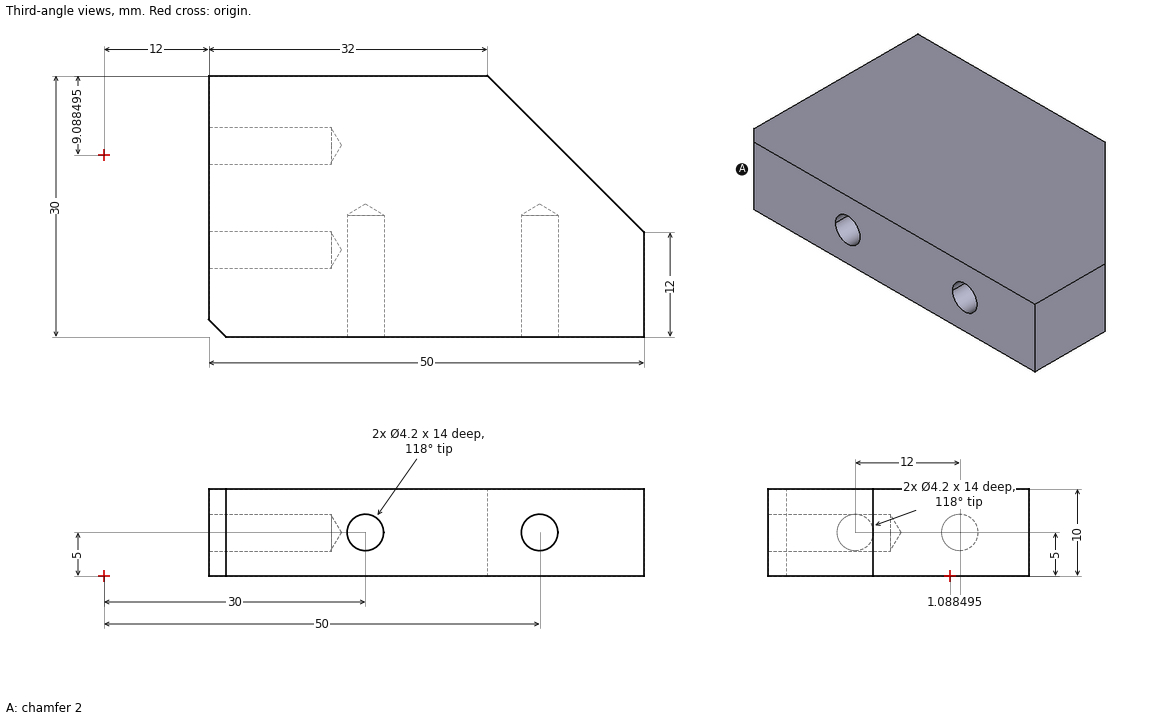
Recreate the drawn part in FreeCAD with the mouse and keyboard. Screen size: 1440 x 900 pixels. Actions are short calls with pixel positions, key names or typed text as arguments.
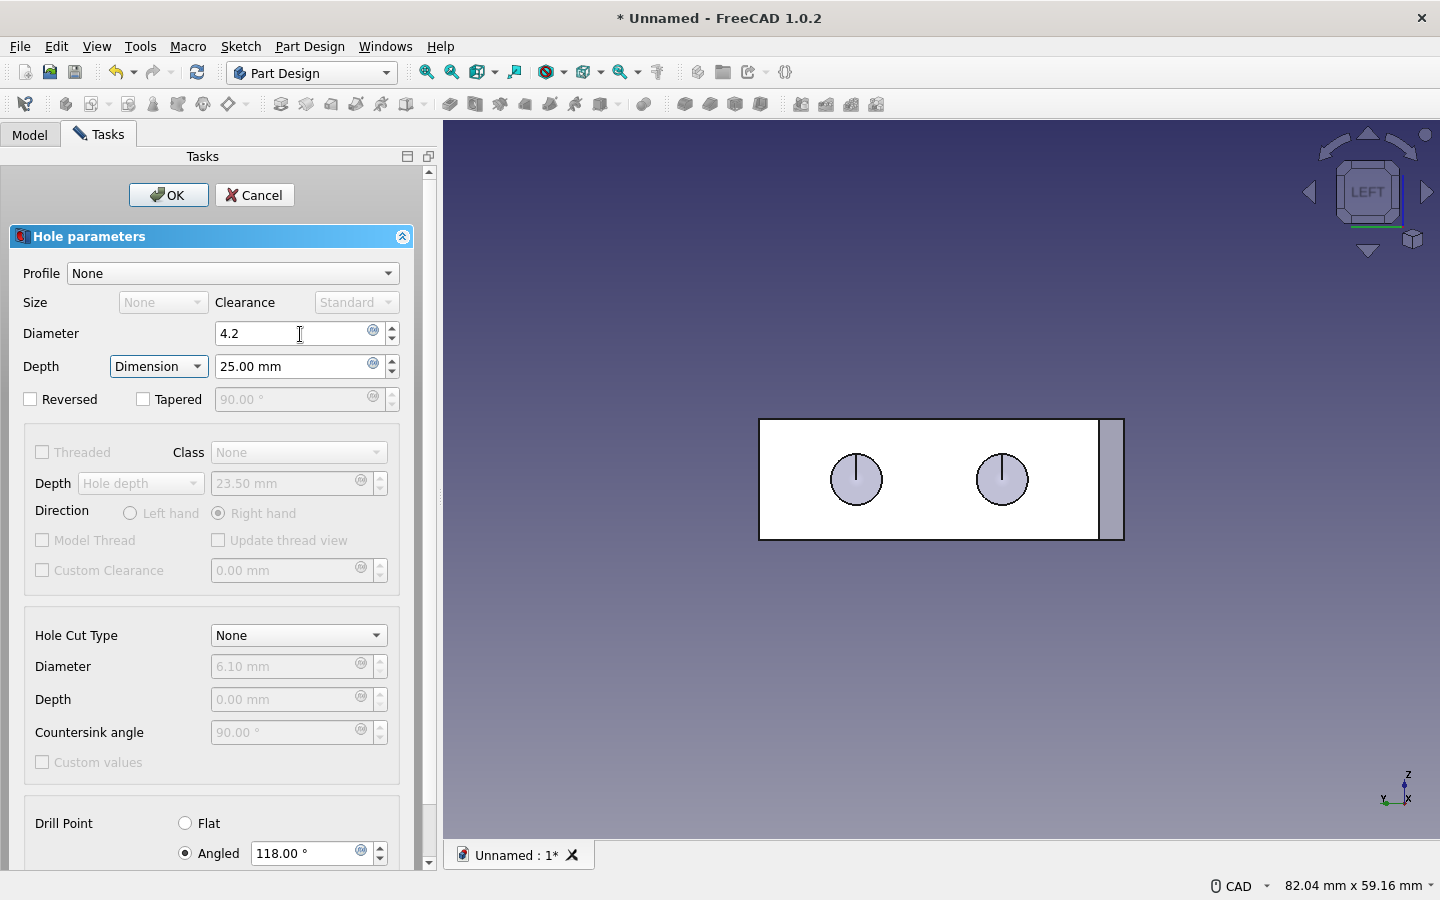
triple_click(300, 366)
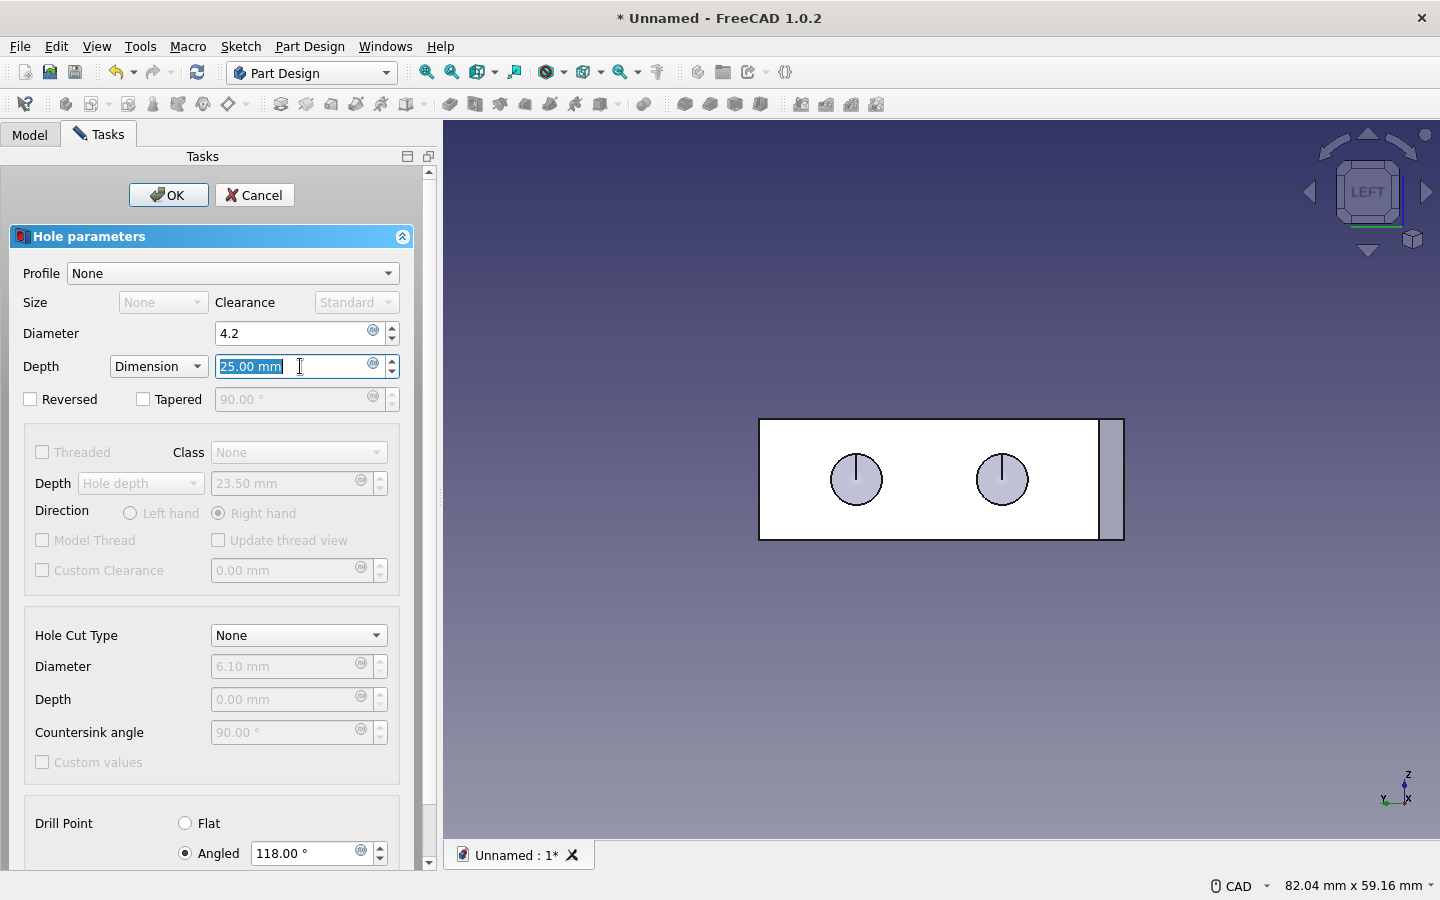
text(14)
key(Tab)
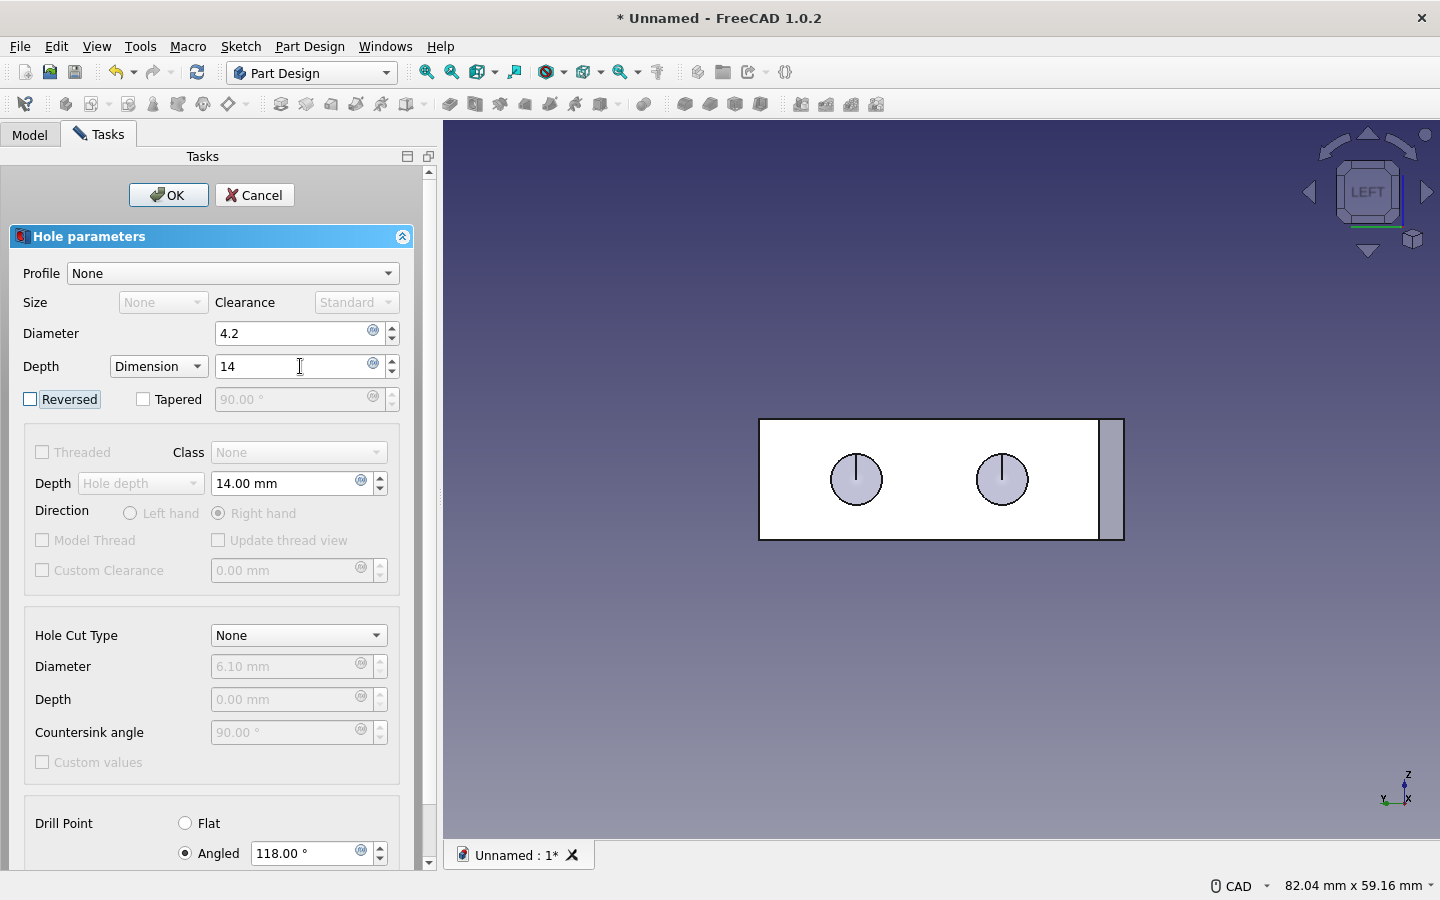
click(169, 195)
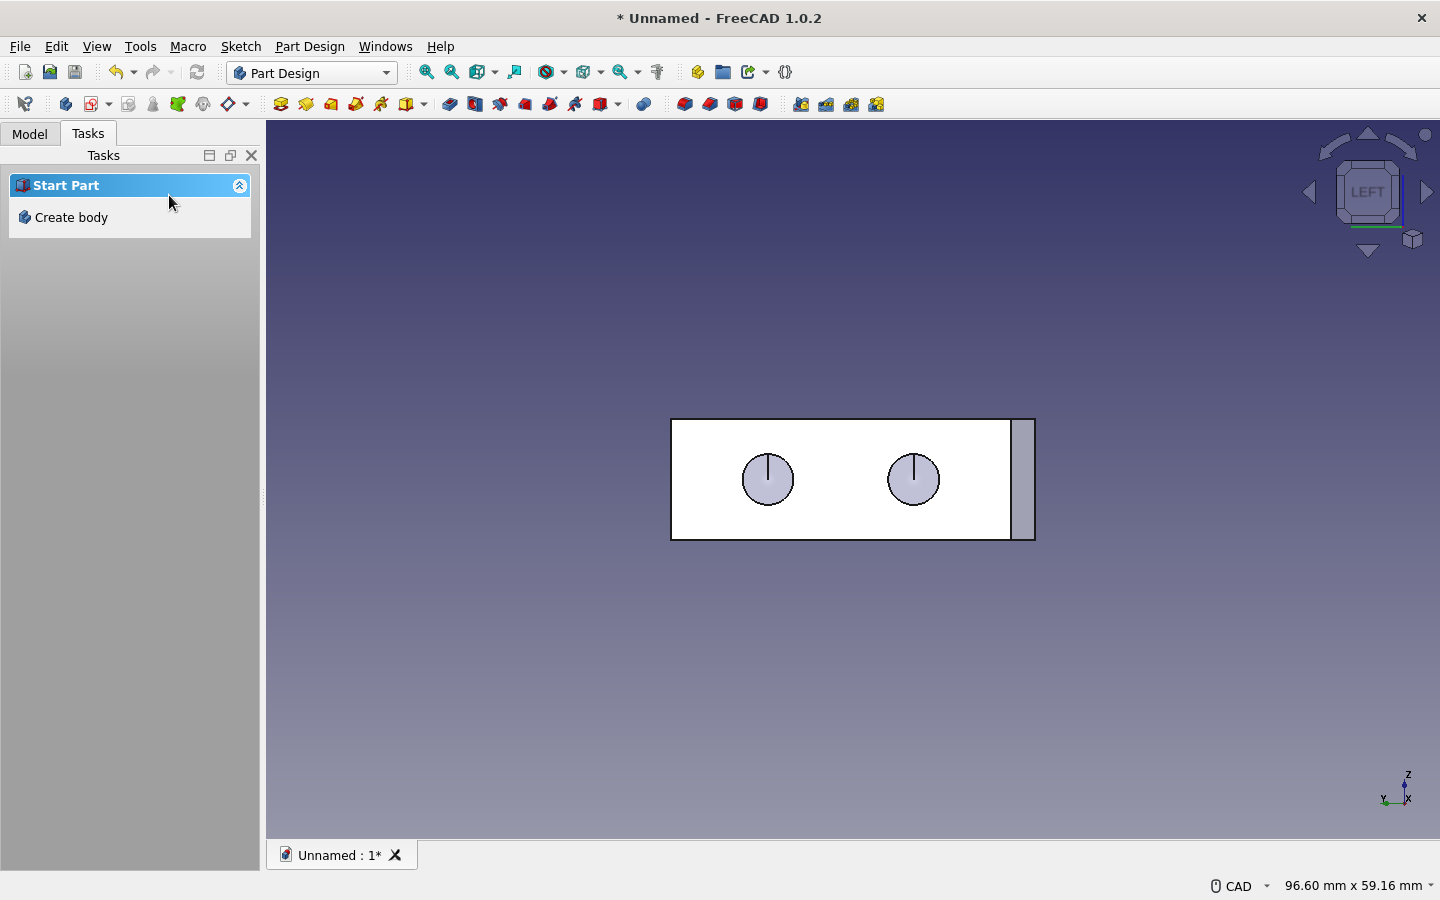
click(427, 72)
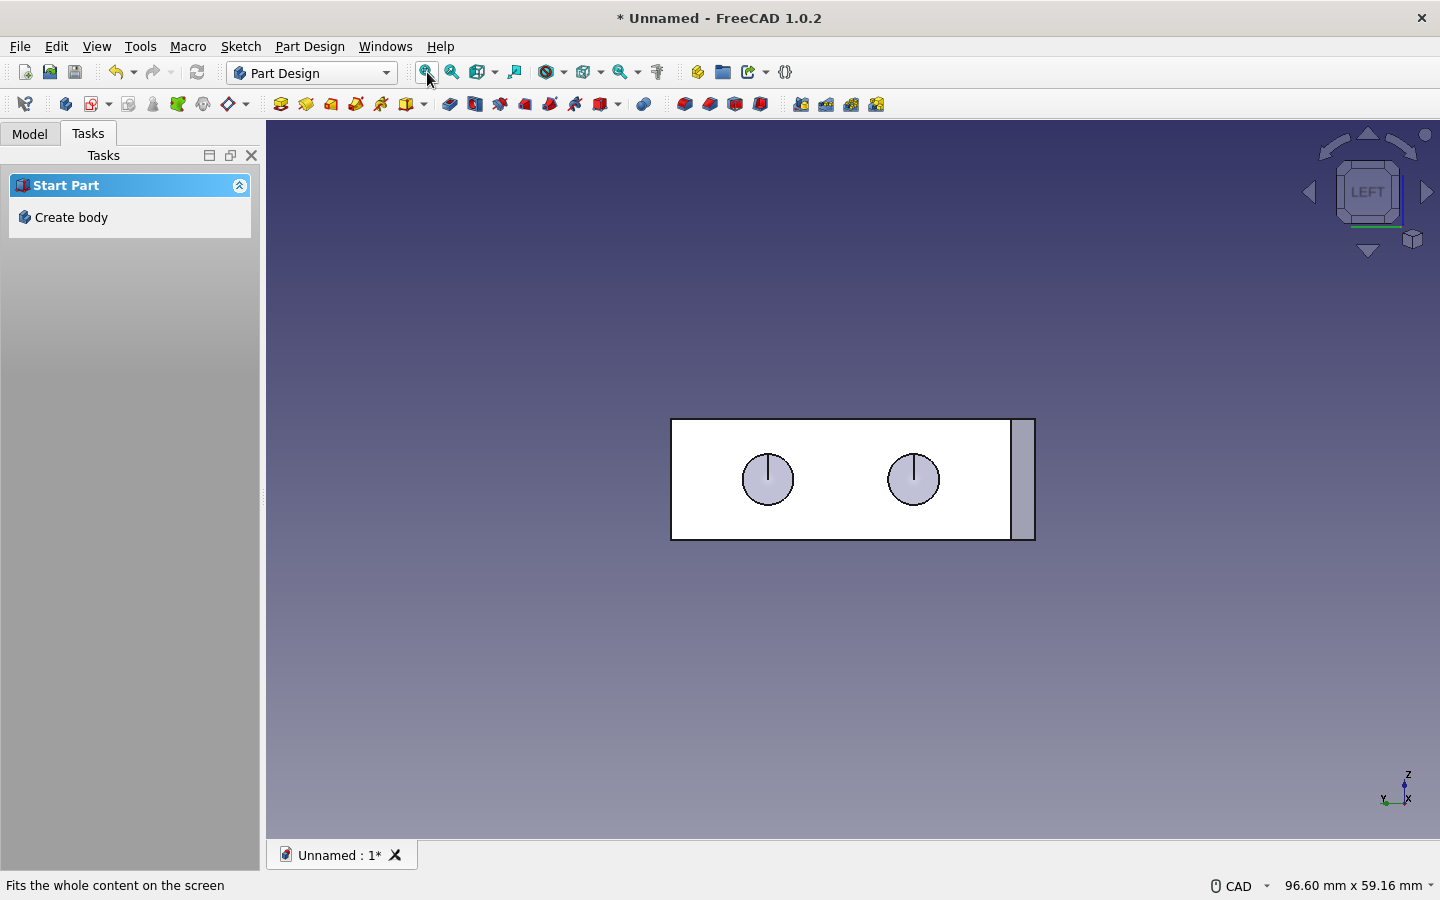
key(0)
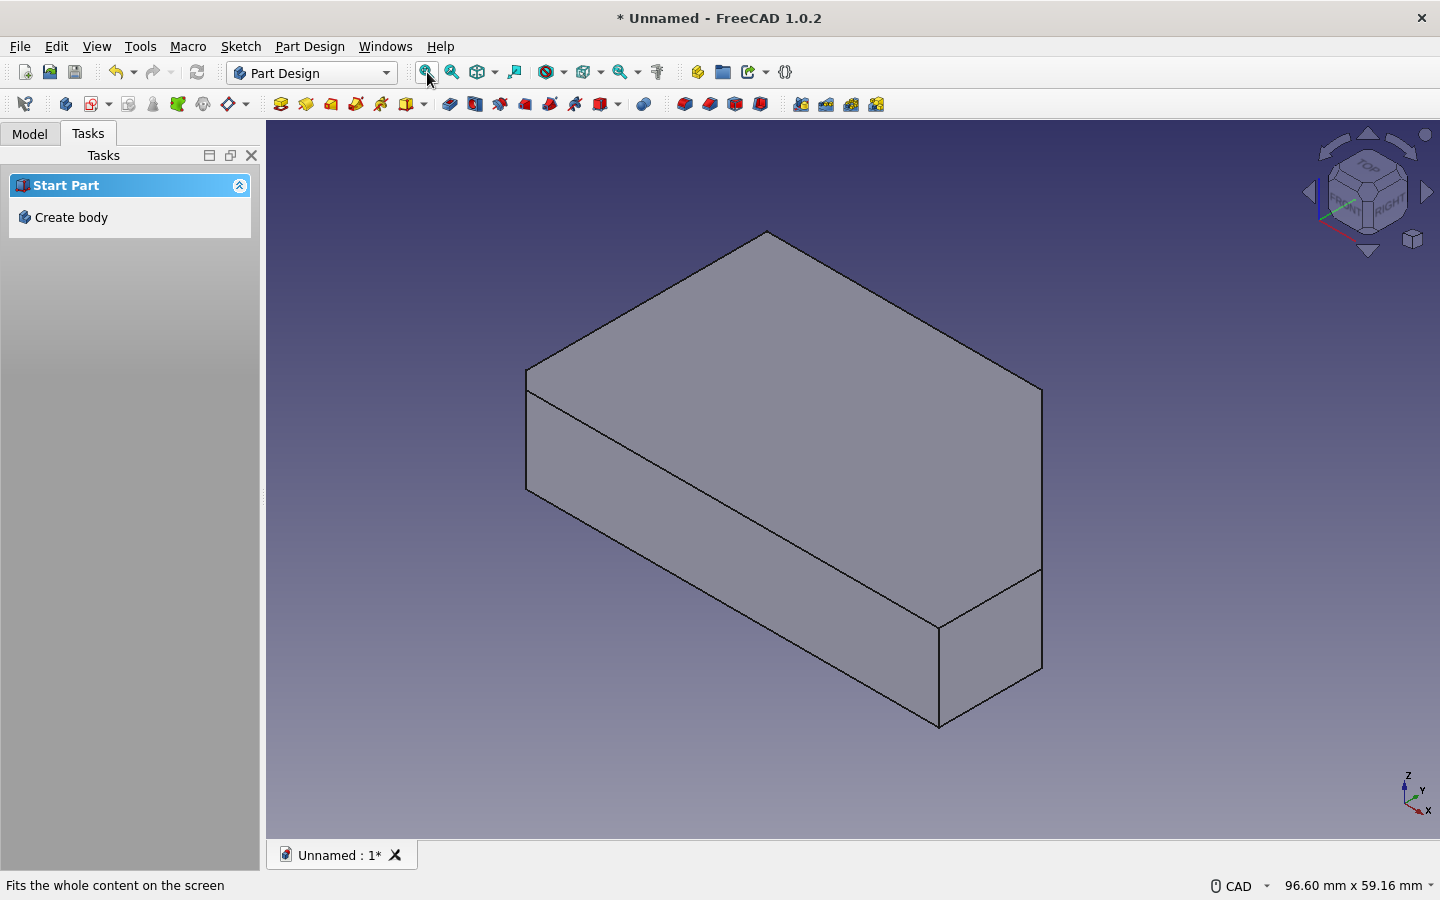
click(851, 626)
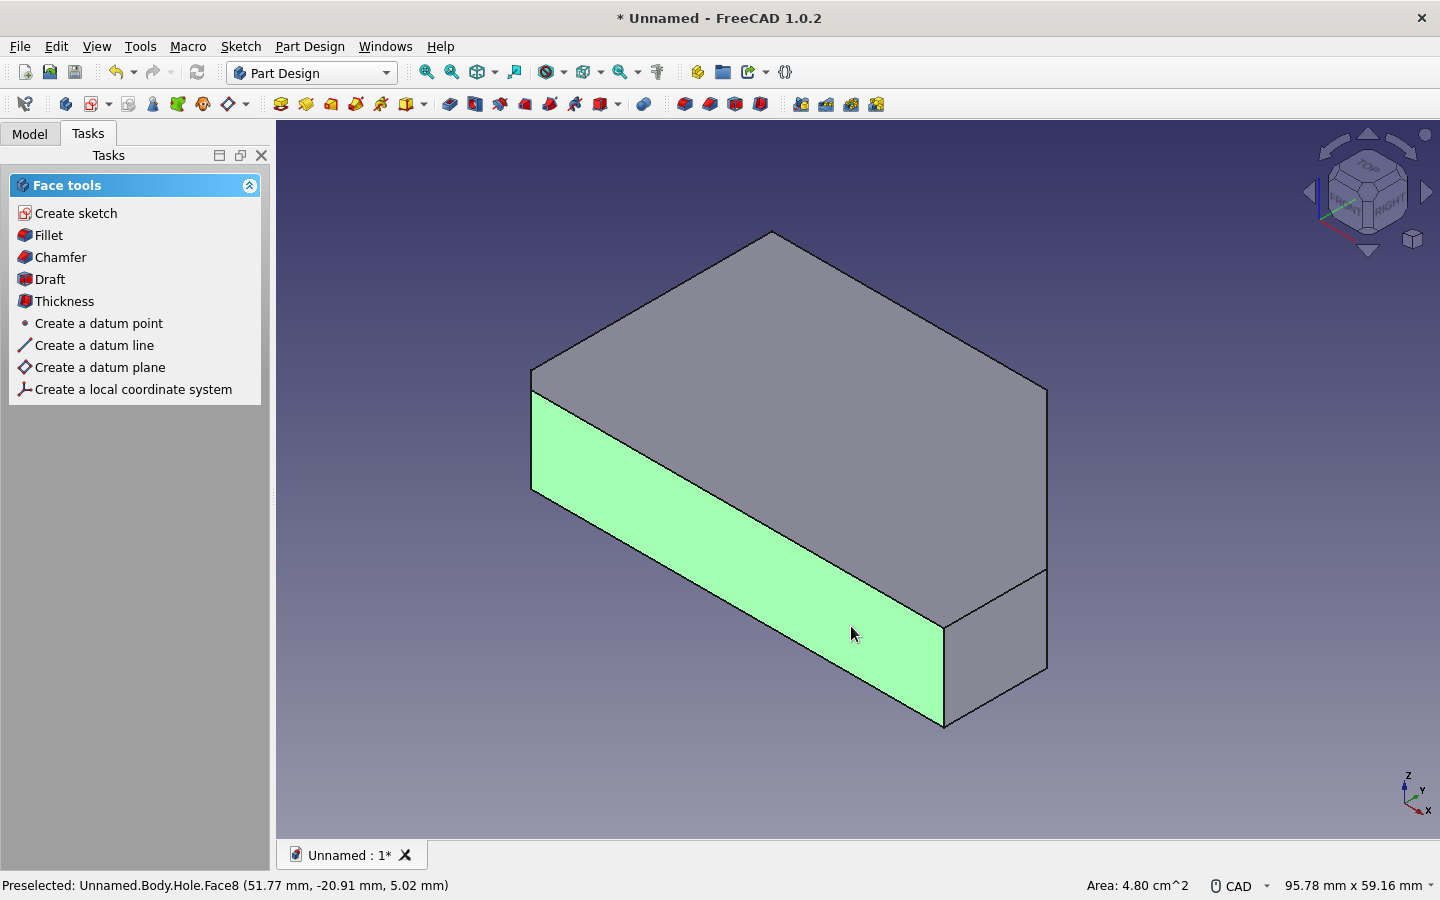
click(90, 104)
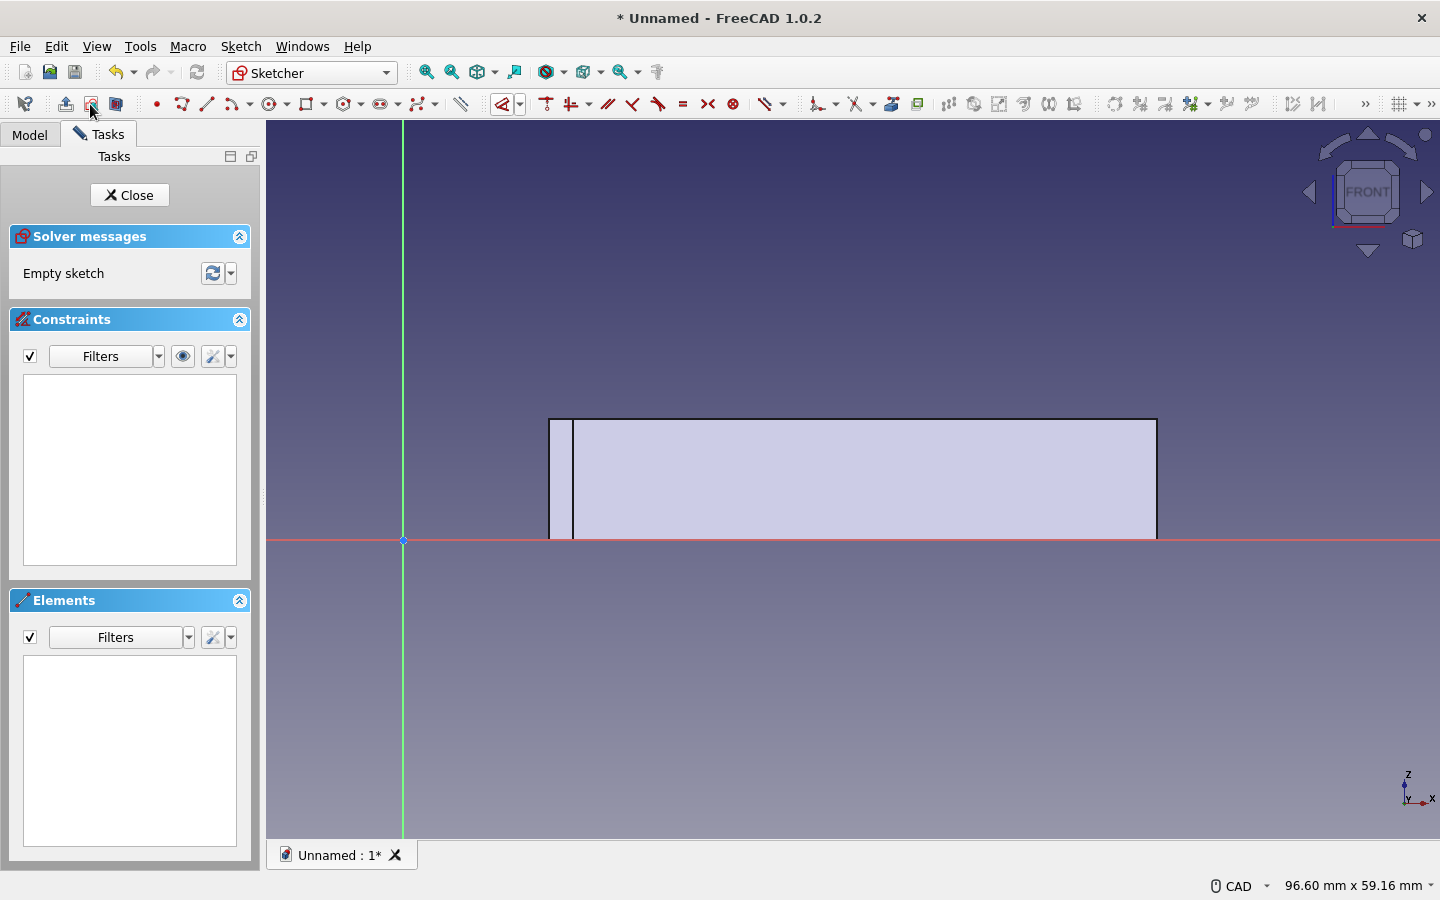
key(g)
key(c)